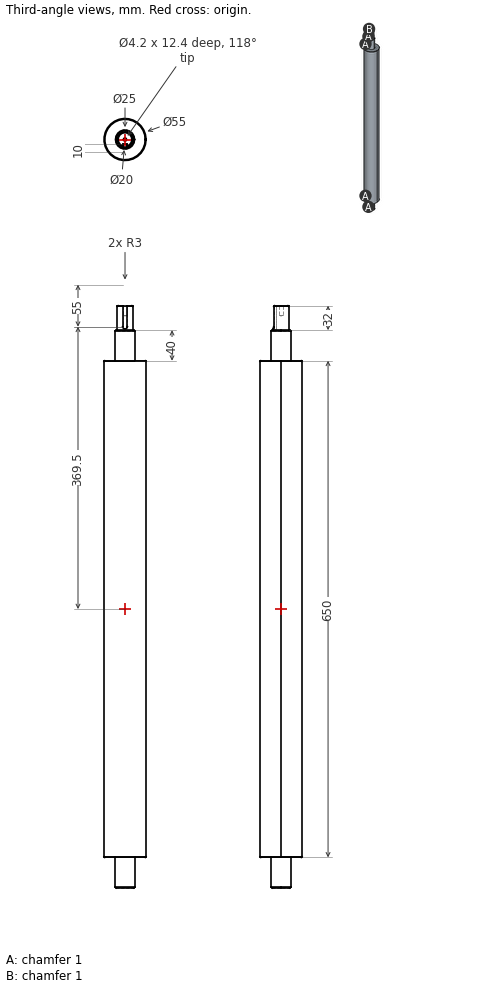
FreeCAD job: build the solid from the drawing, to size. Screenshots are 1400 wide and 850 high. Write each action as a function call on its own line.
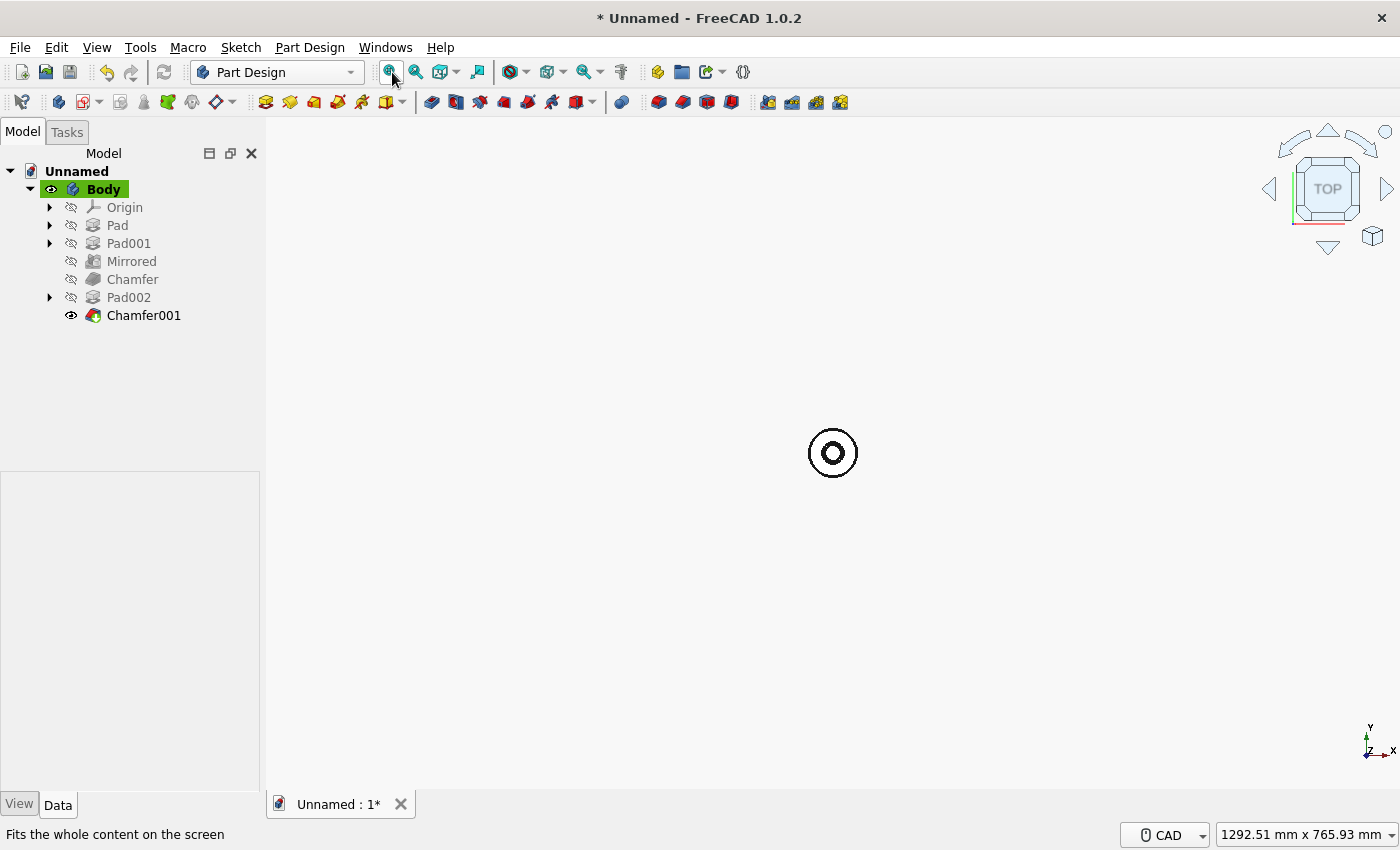
click(50, 207)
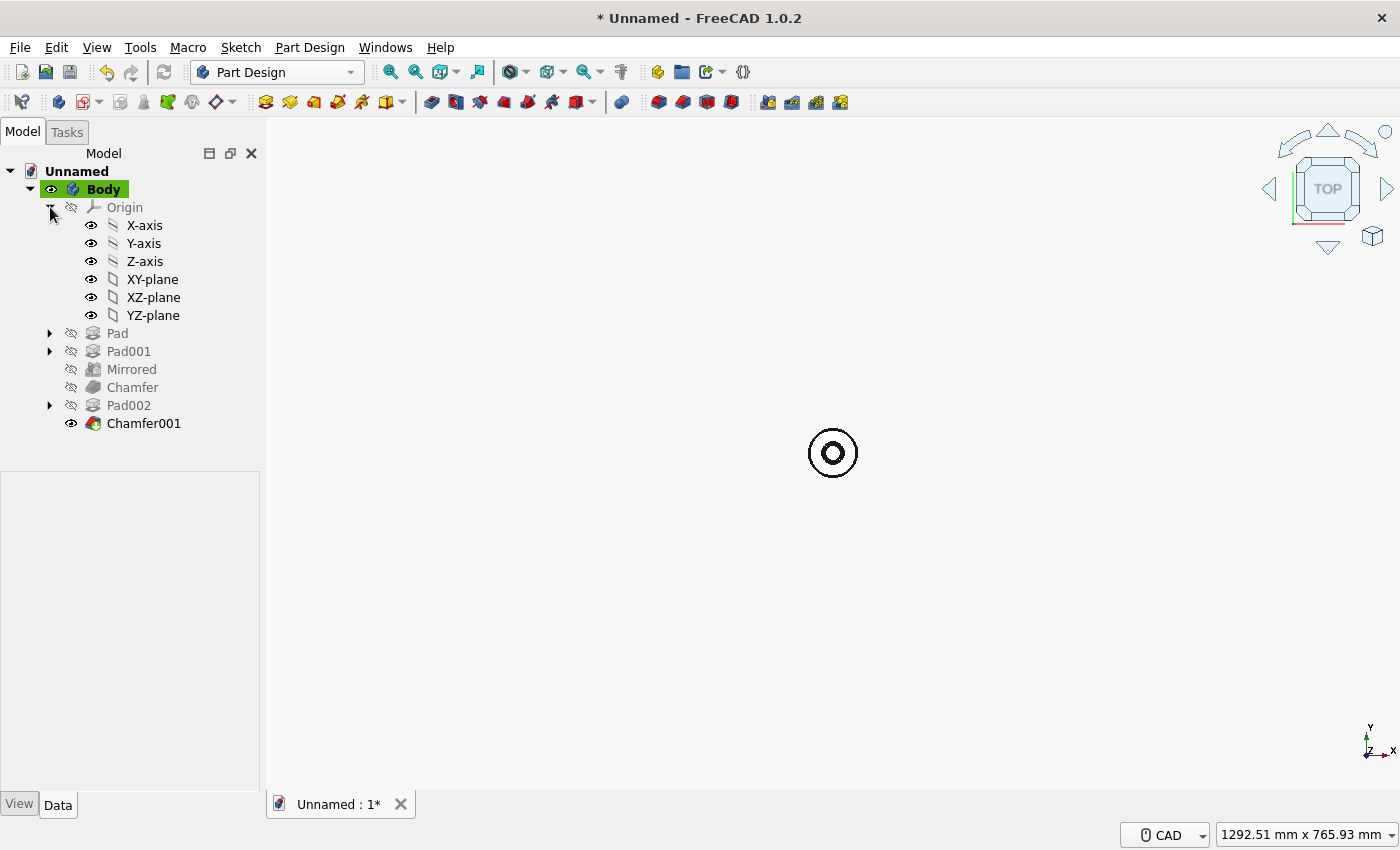
click(136, 297)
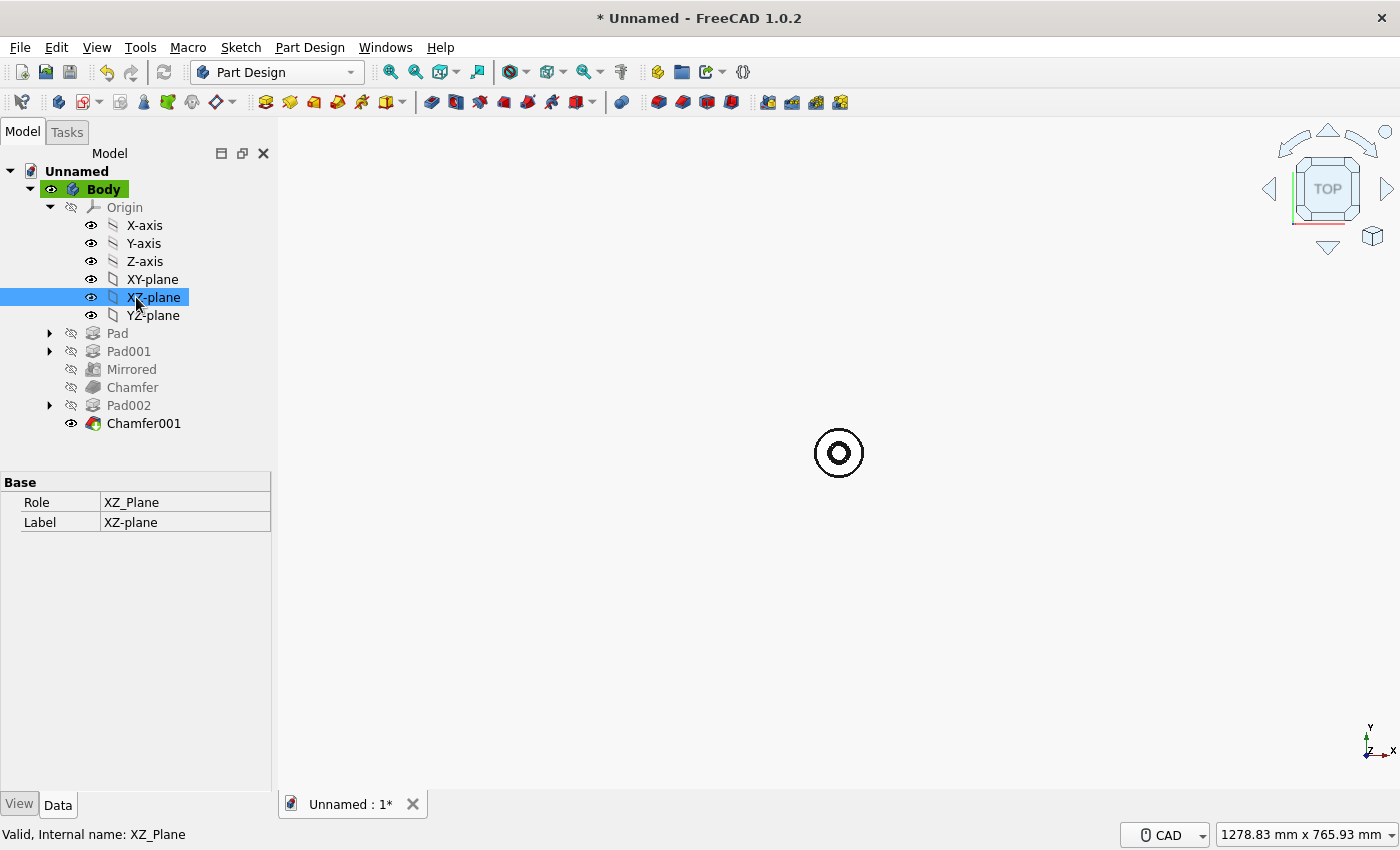
click(216, 102)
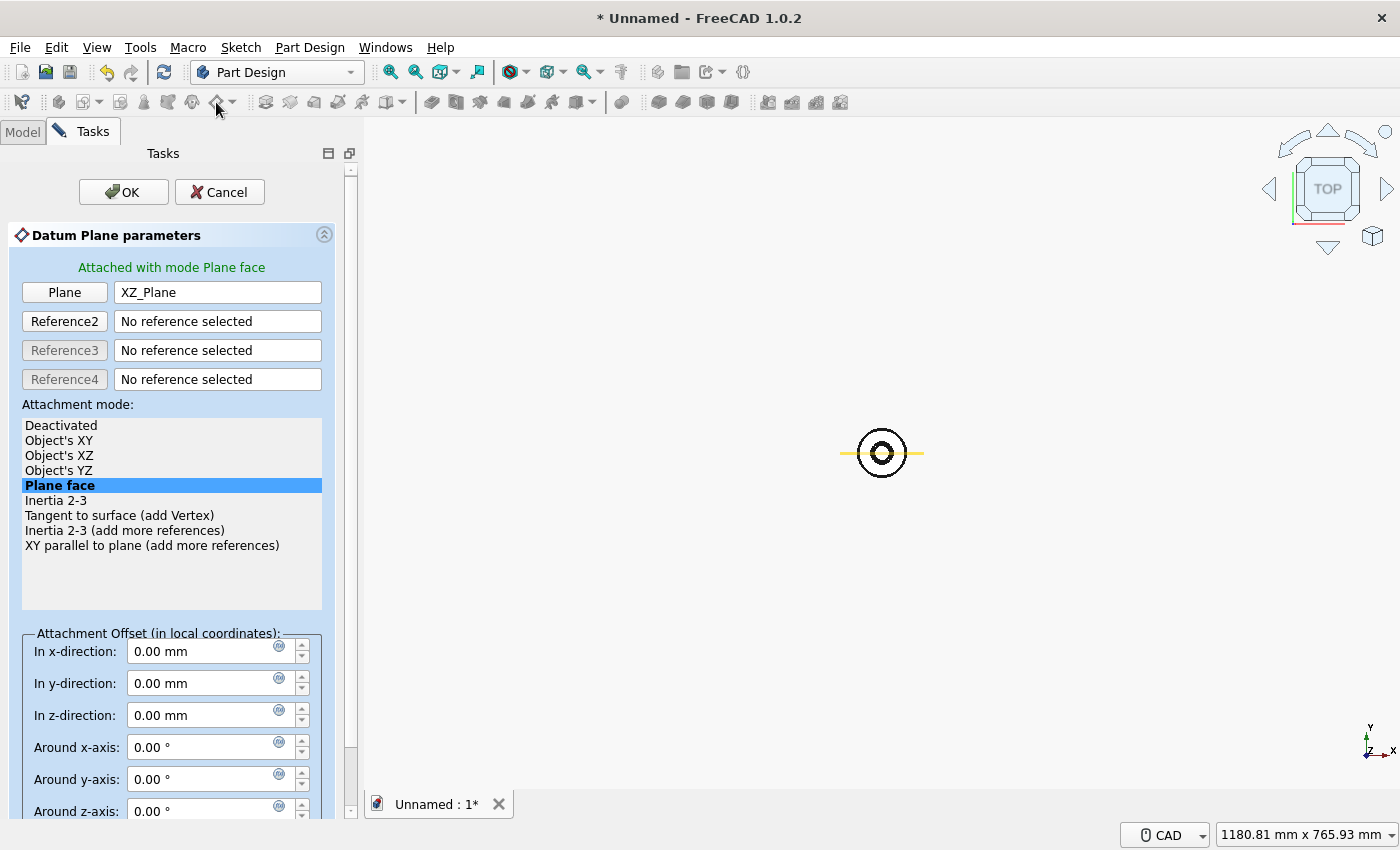
triple_click(210, 715)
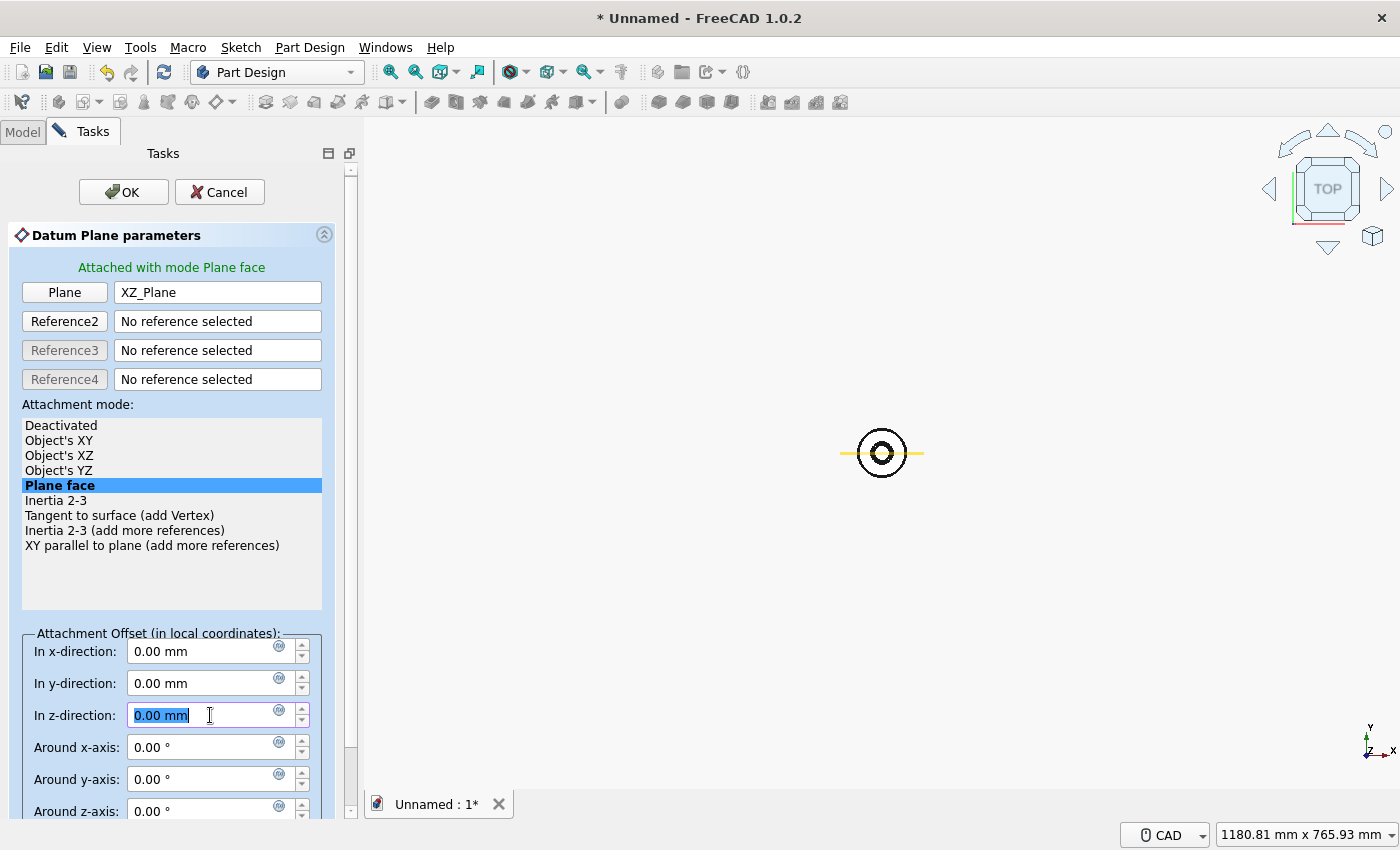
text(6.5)
key(Tab)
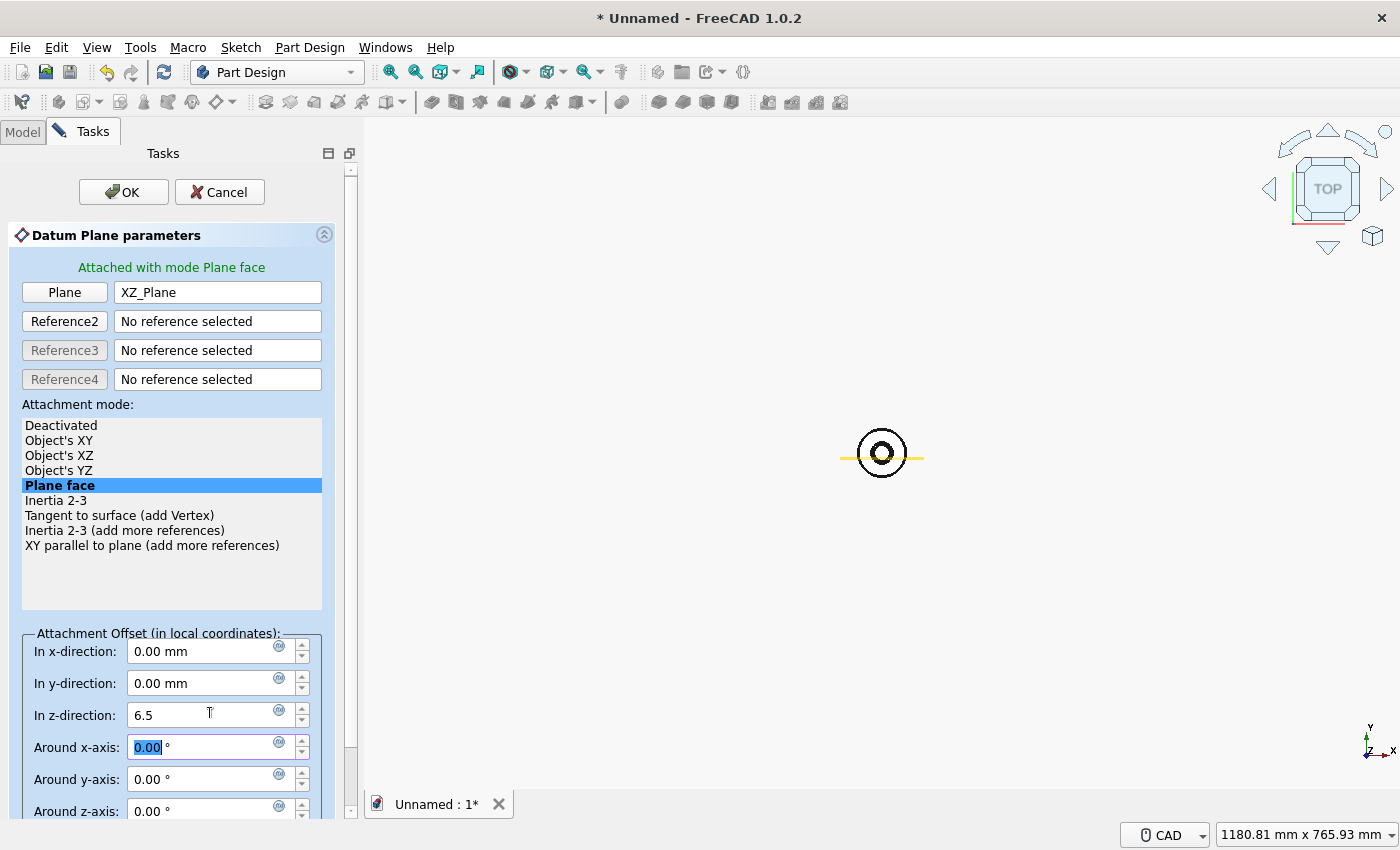
click(124, 192)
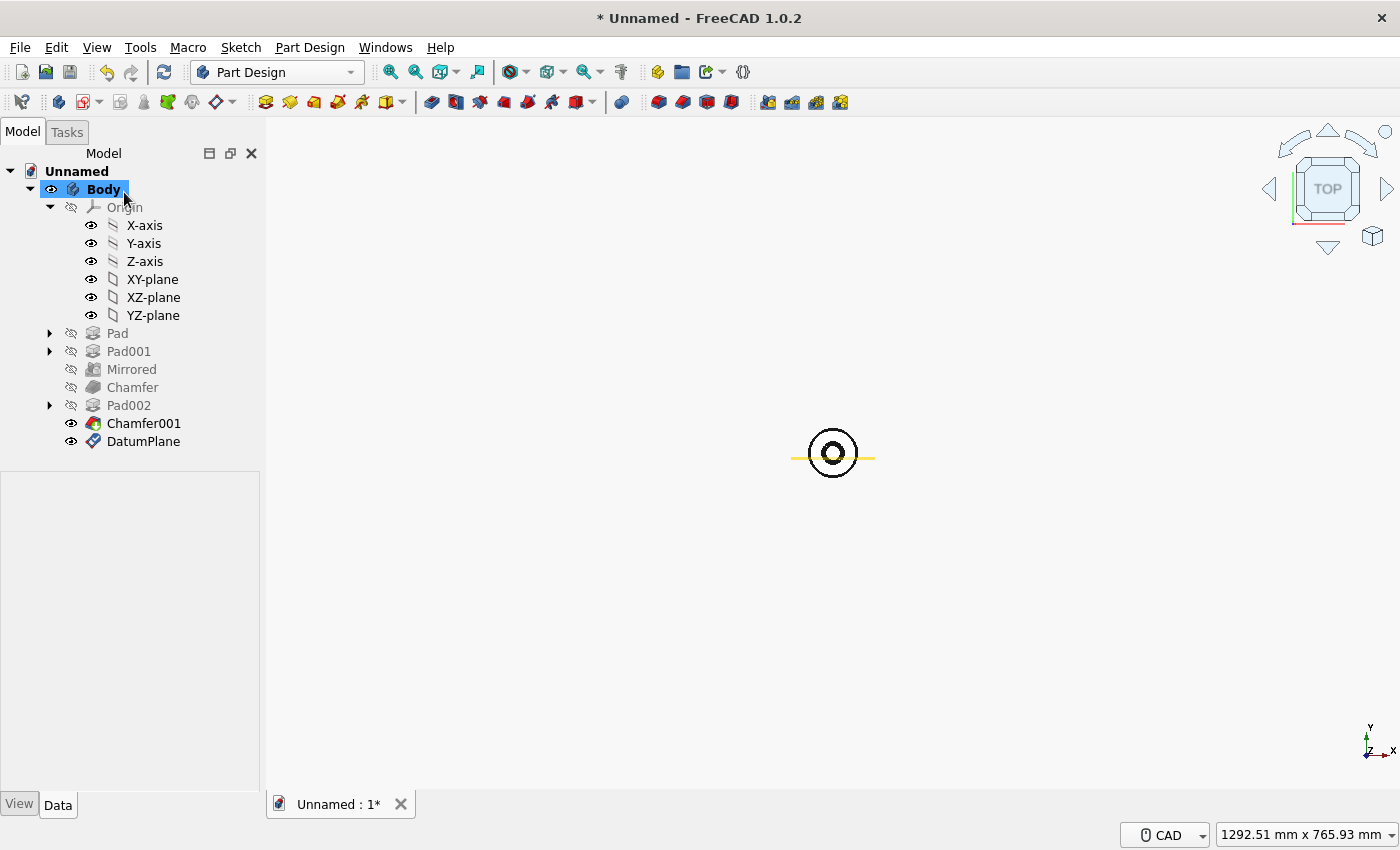
click(116, 441)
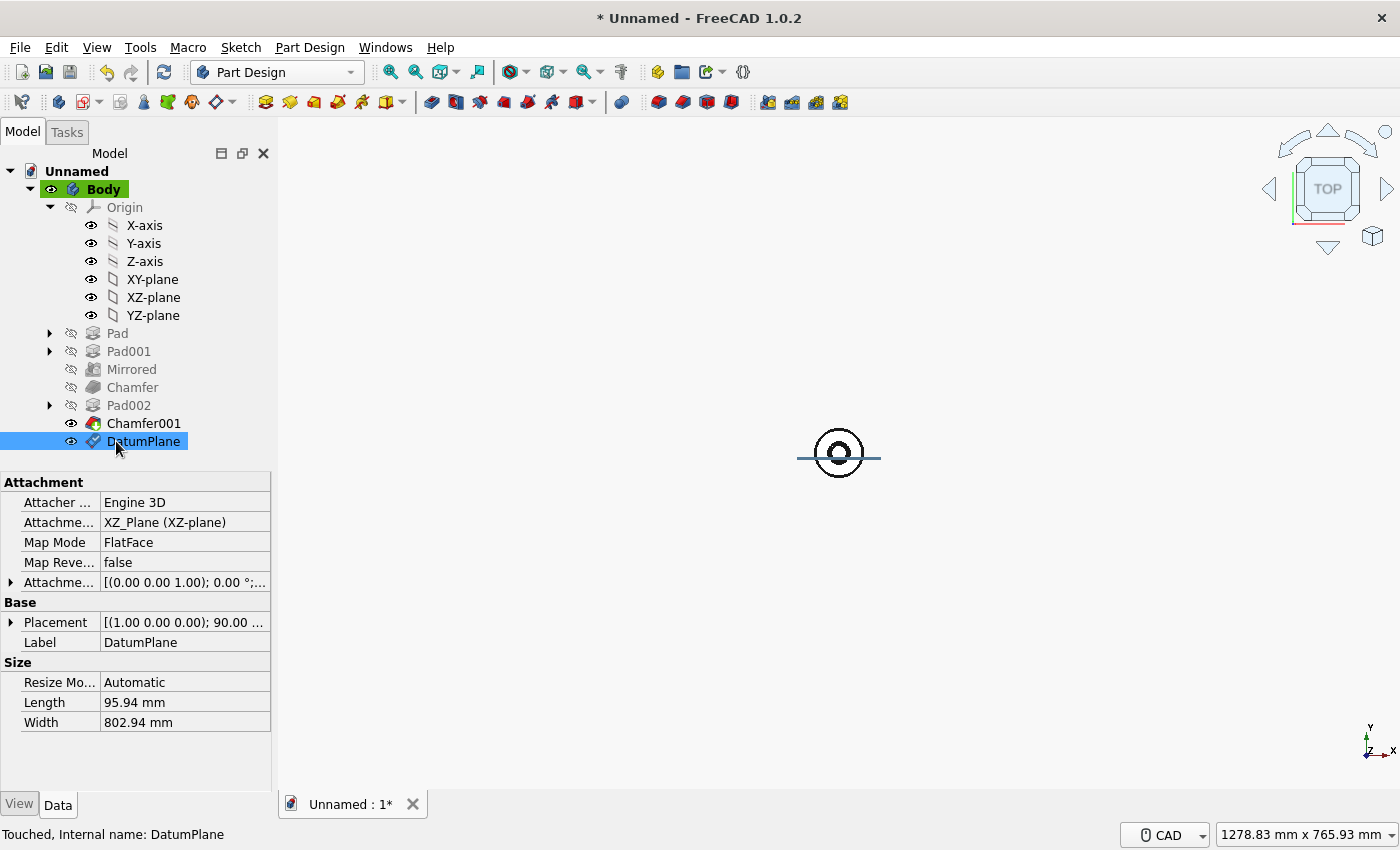
click(84, 102)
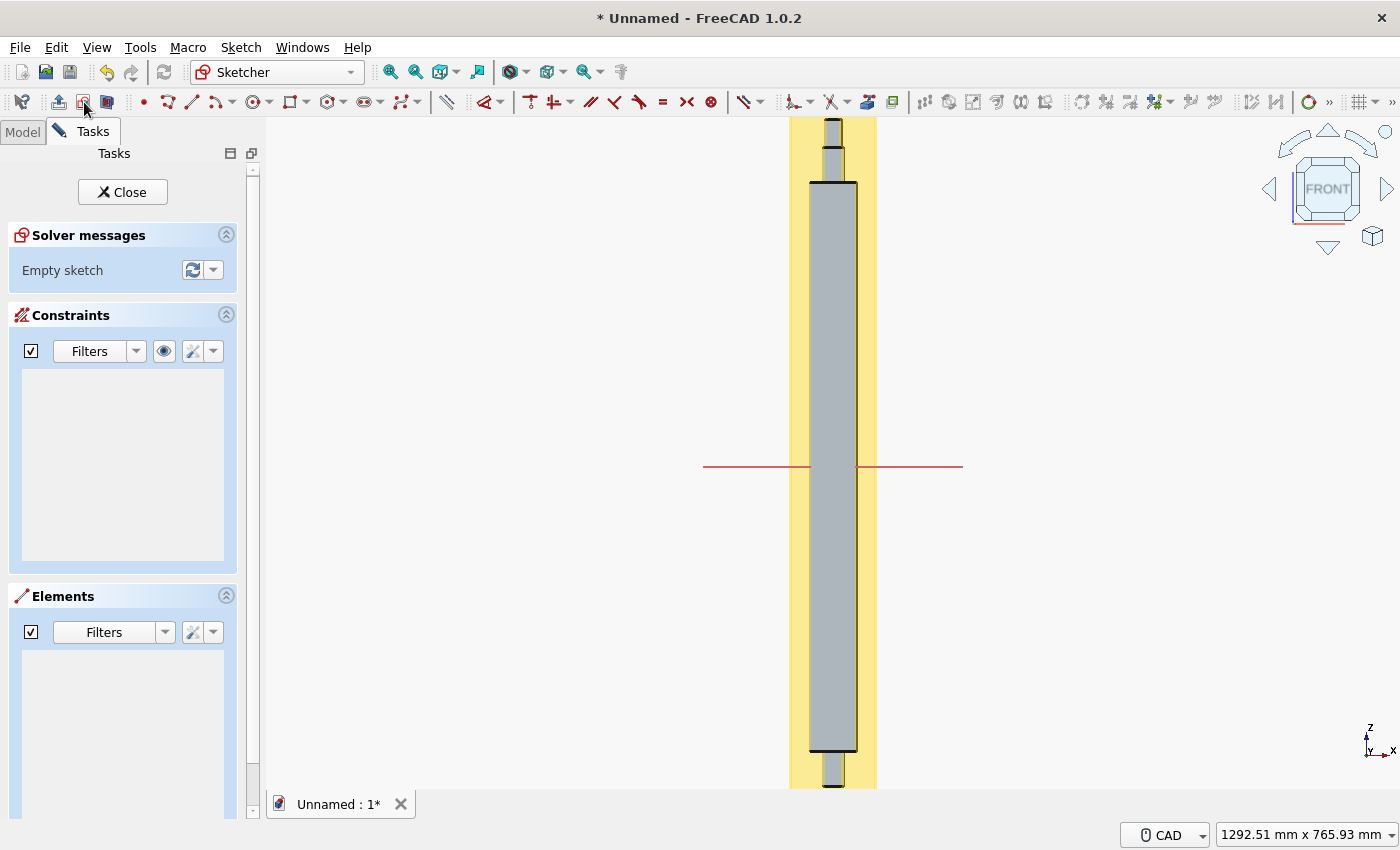
click(108, 102)